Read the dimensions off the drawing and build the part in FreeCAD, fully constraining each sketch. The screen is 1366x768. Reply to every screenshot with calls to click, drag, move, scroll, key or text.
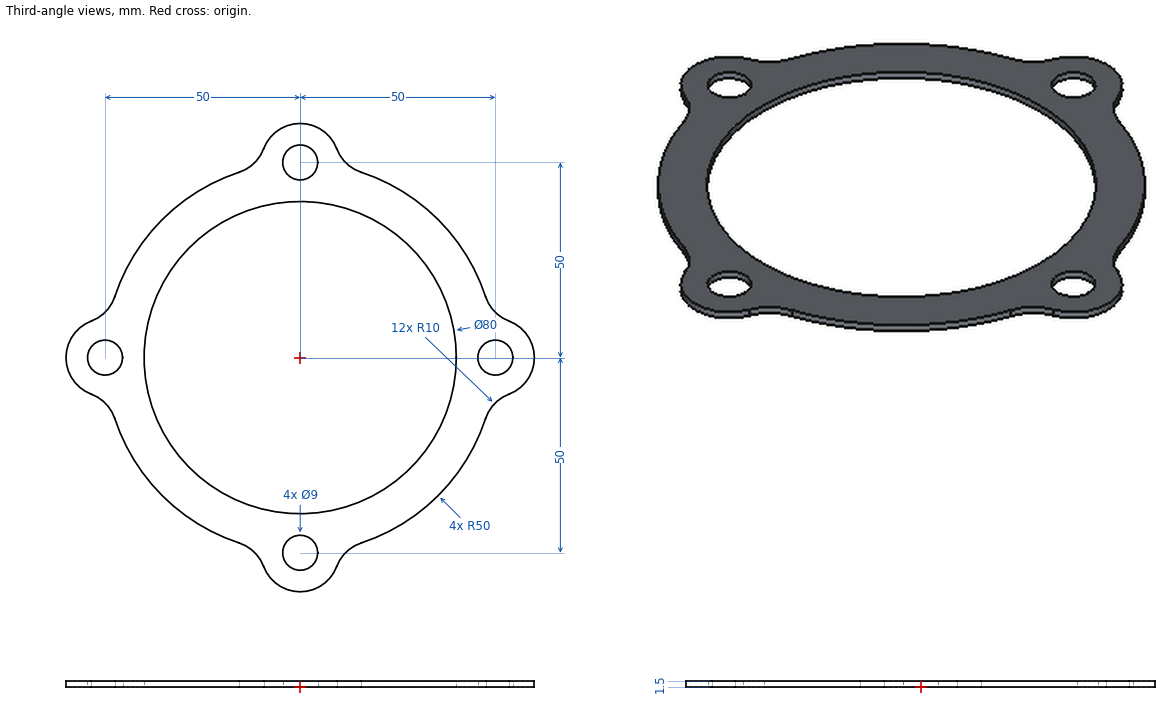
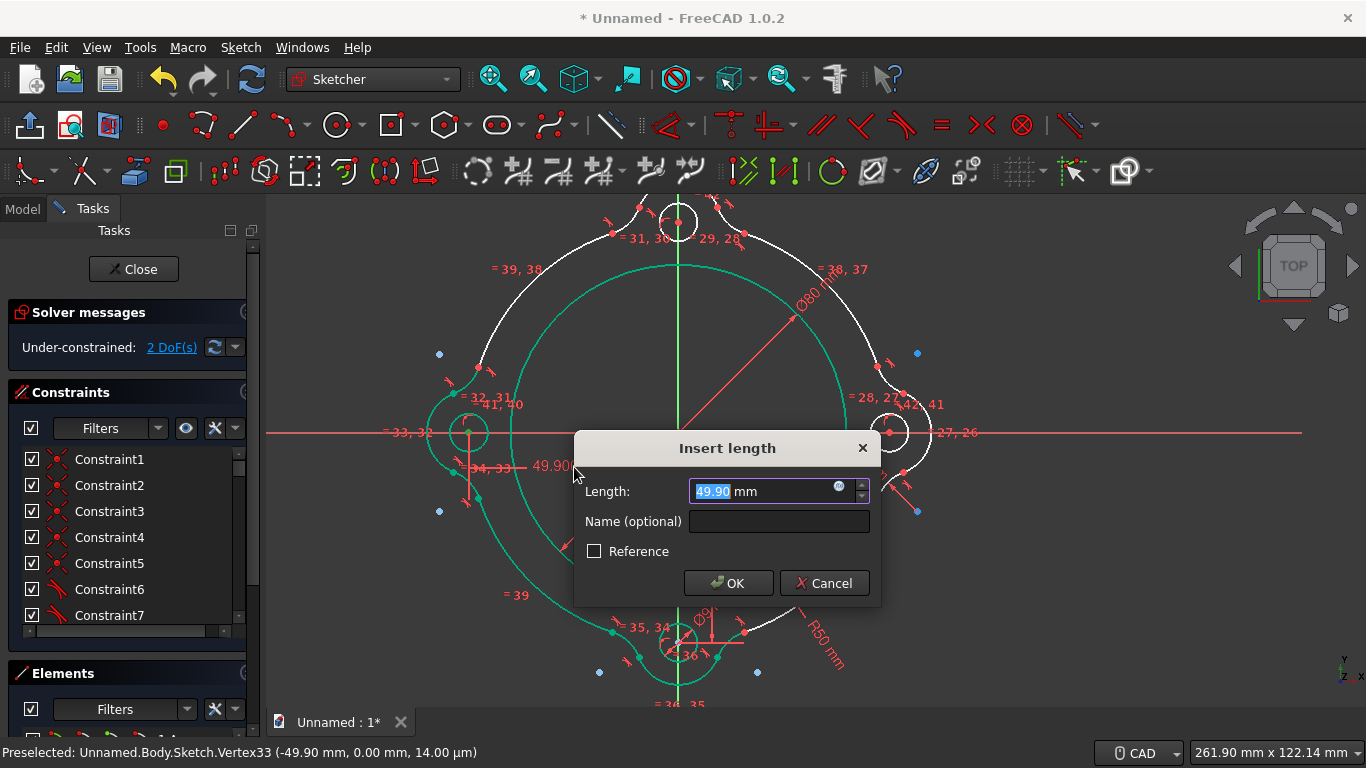
text(50)
key(Return)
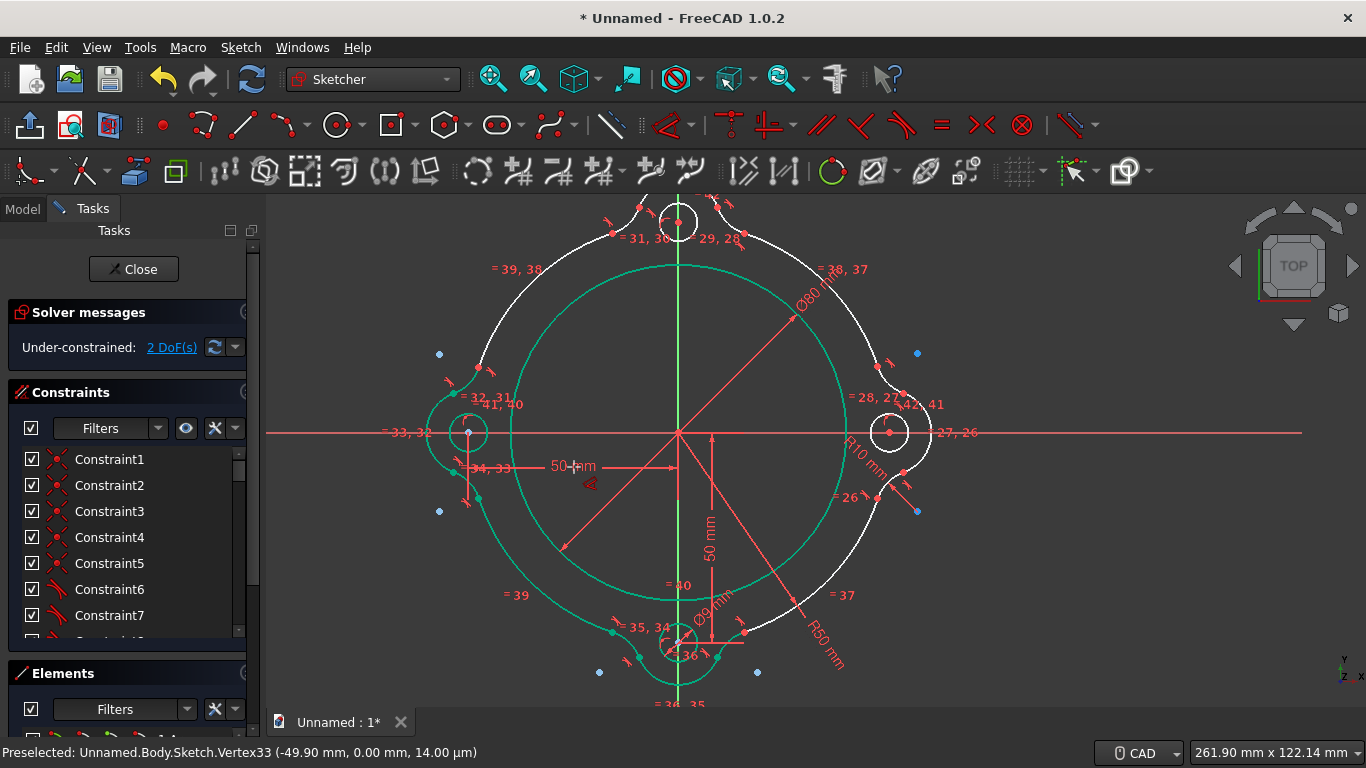
click(889, 433)
click(784, 467)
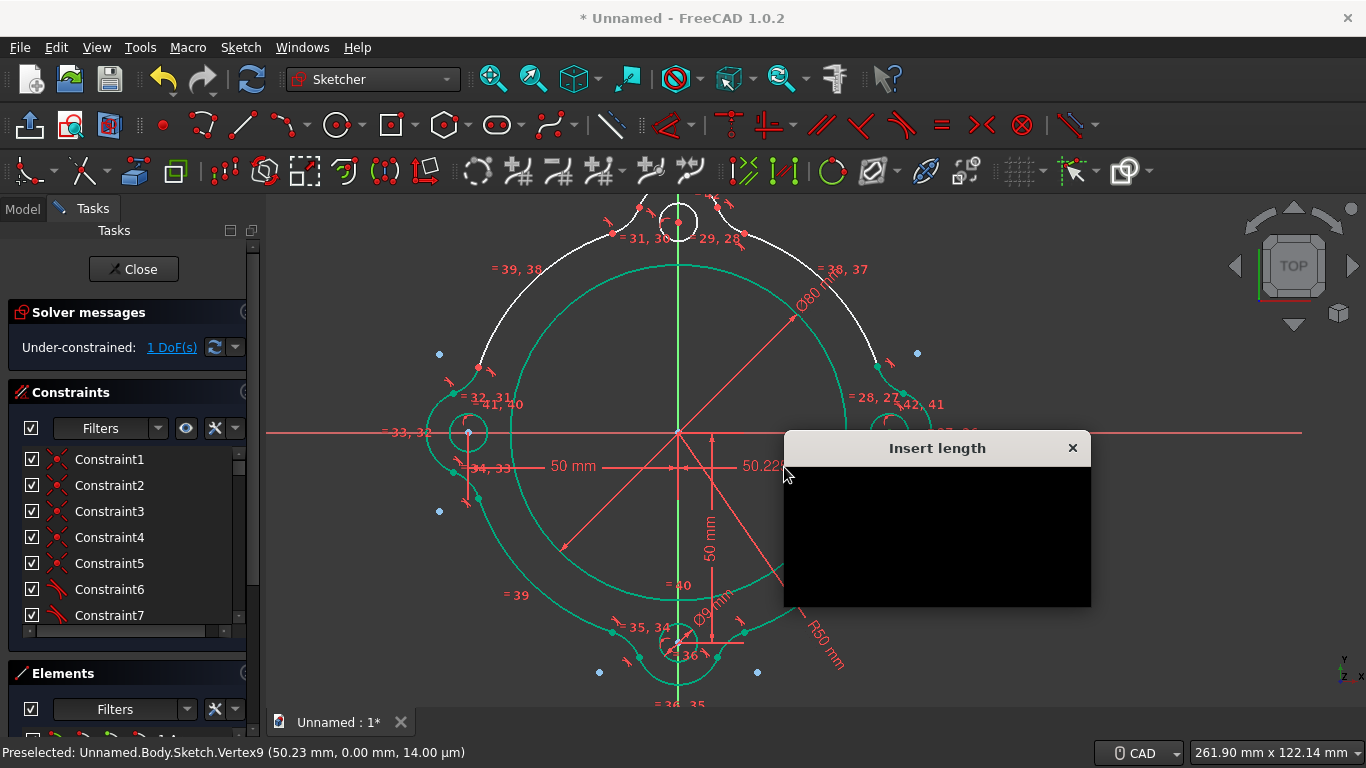
text(50)
key(Return)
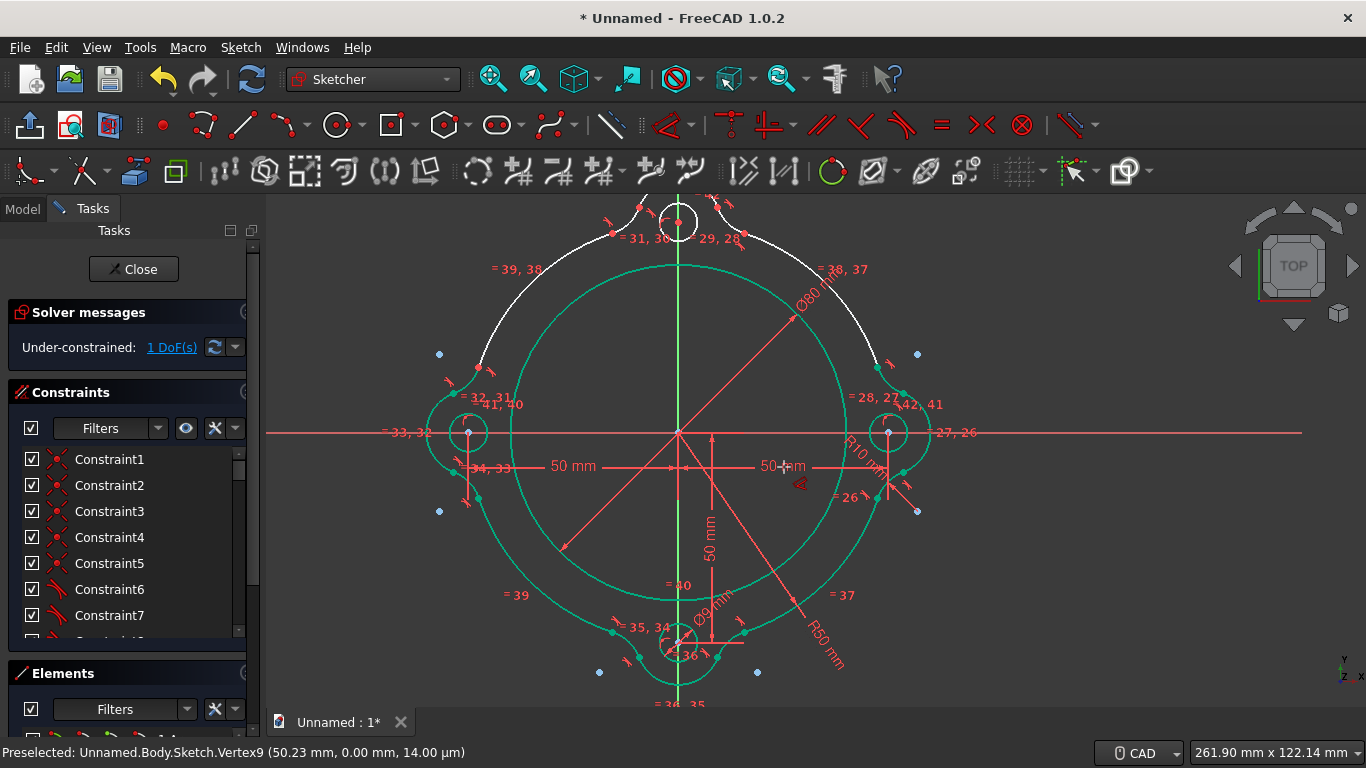
click(678, 222)
click(712, 328)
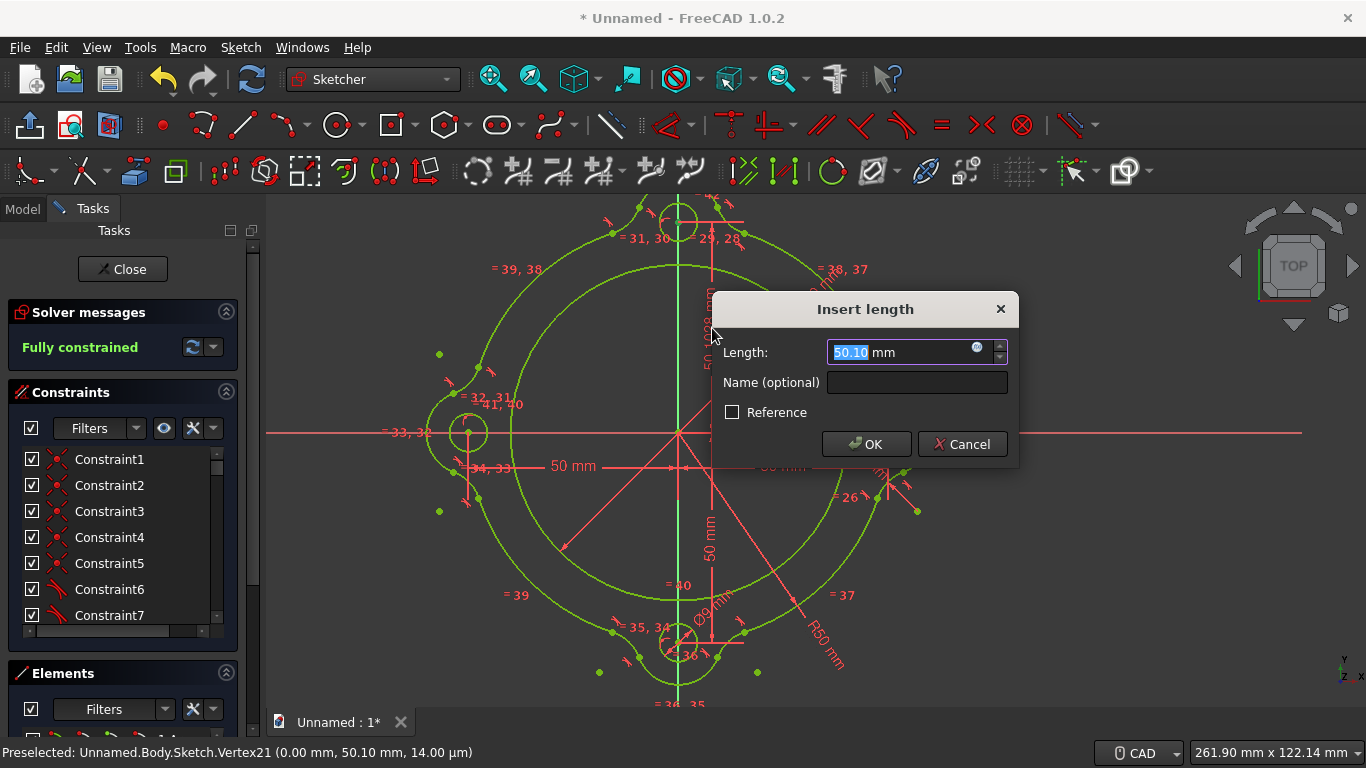
text(50)
key(Return)
key(Escape)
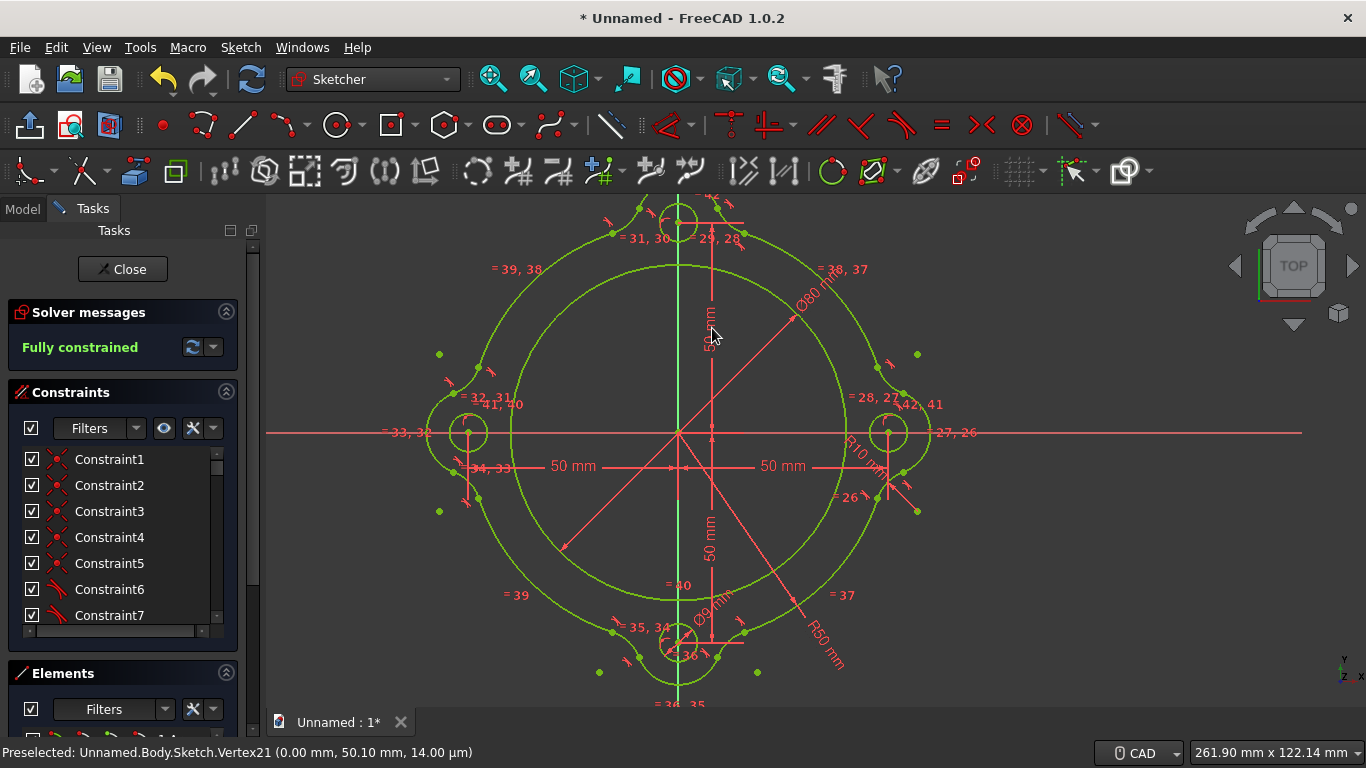
click(123, 269)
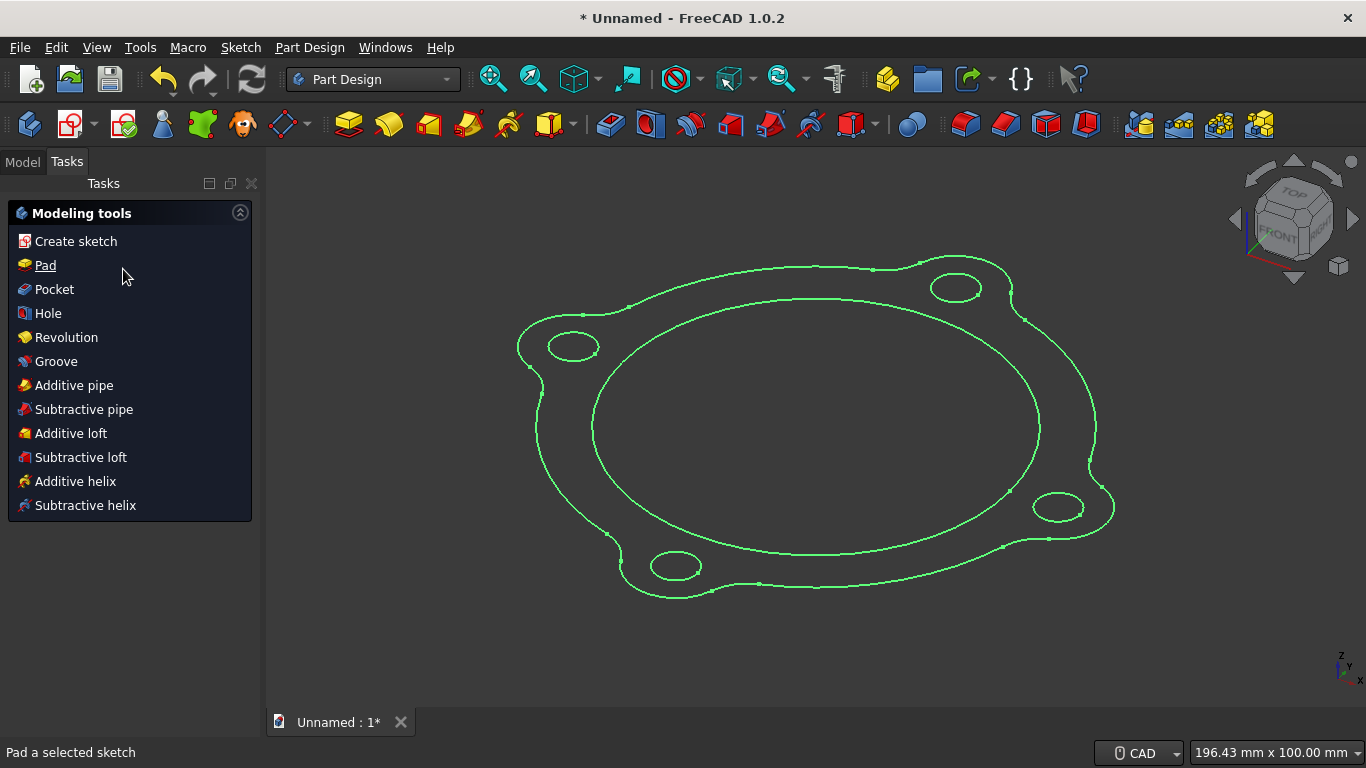
click(350, 124)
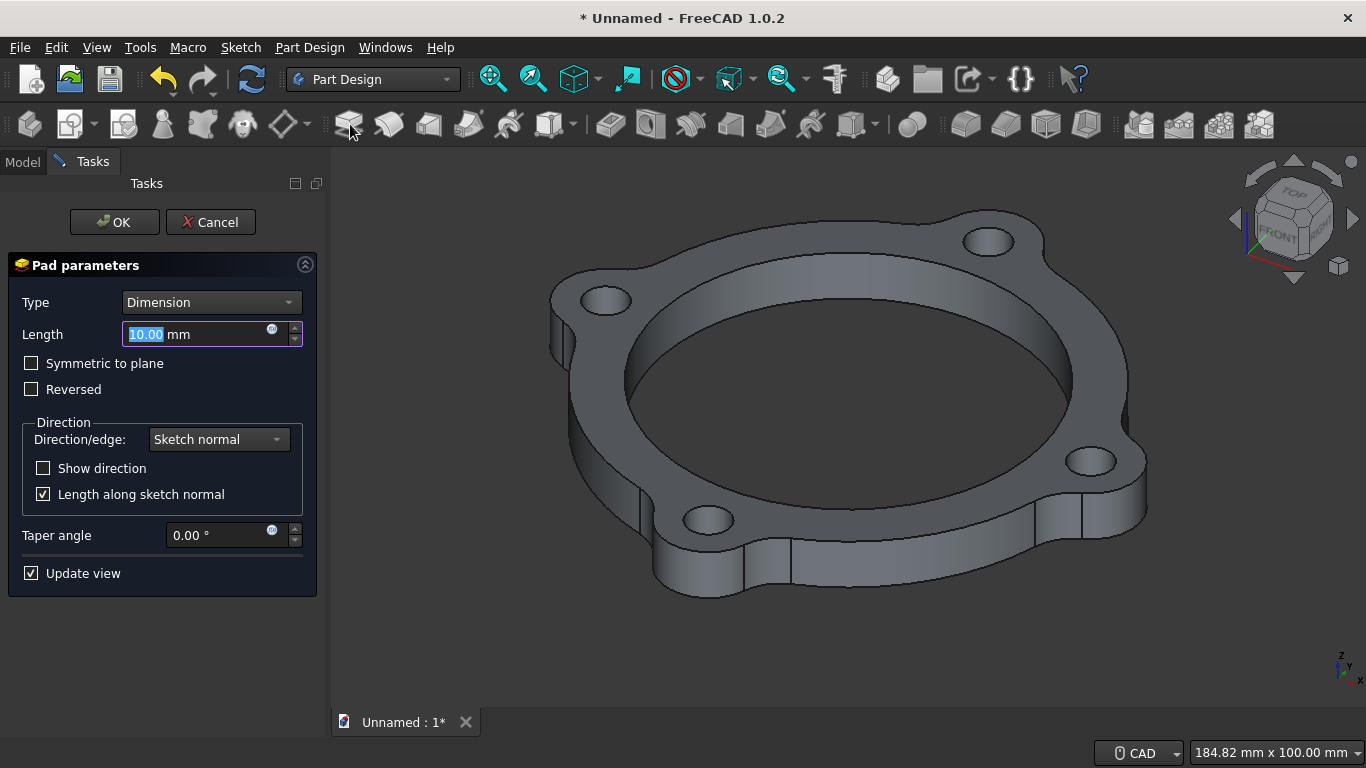
text(1.5)
key(Tab)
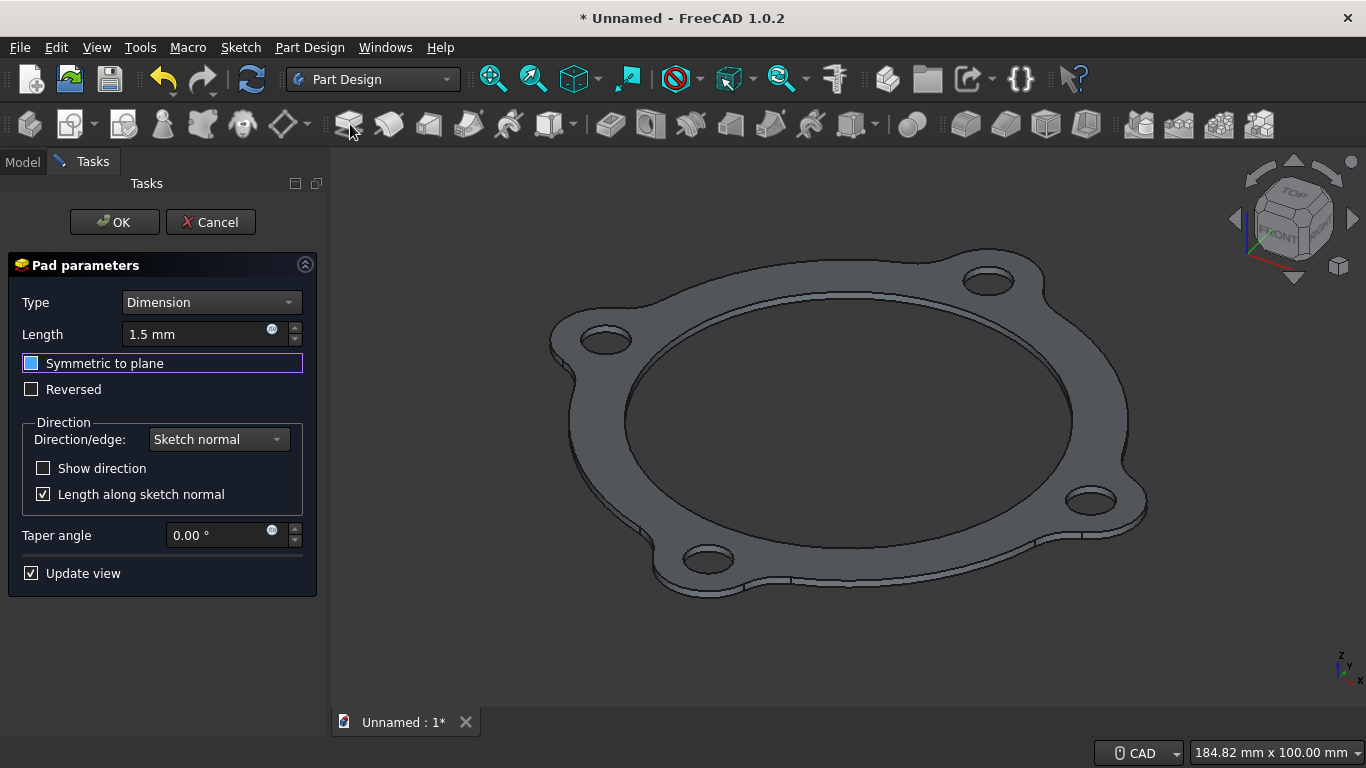
click(115, 222)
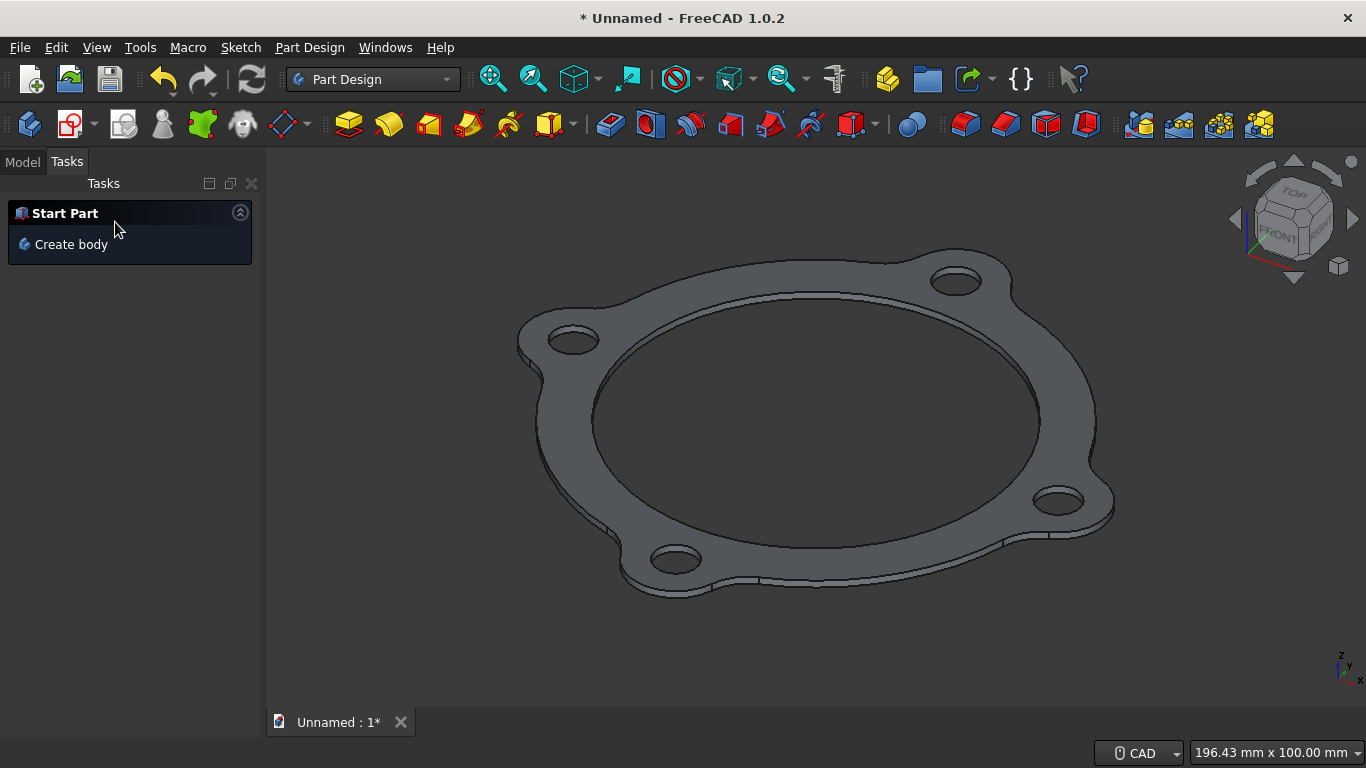
key(0)